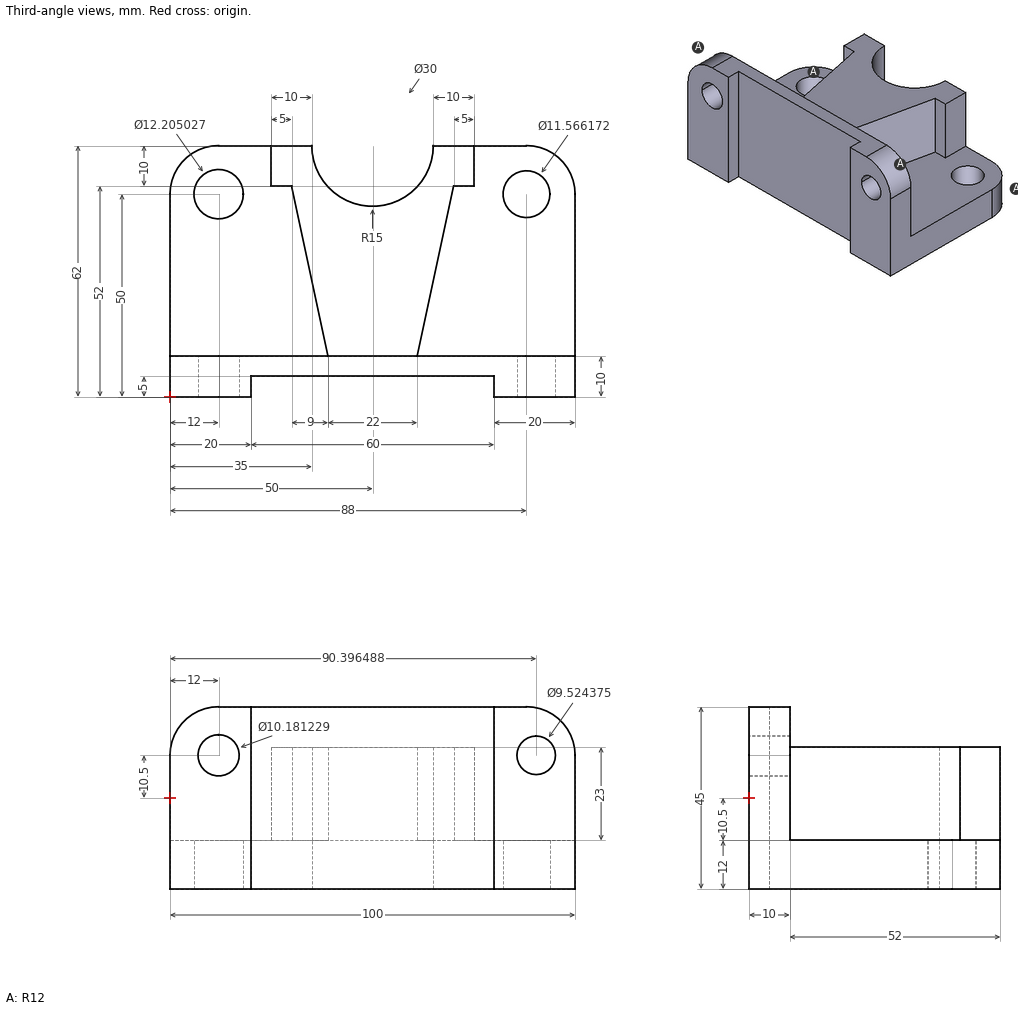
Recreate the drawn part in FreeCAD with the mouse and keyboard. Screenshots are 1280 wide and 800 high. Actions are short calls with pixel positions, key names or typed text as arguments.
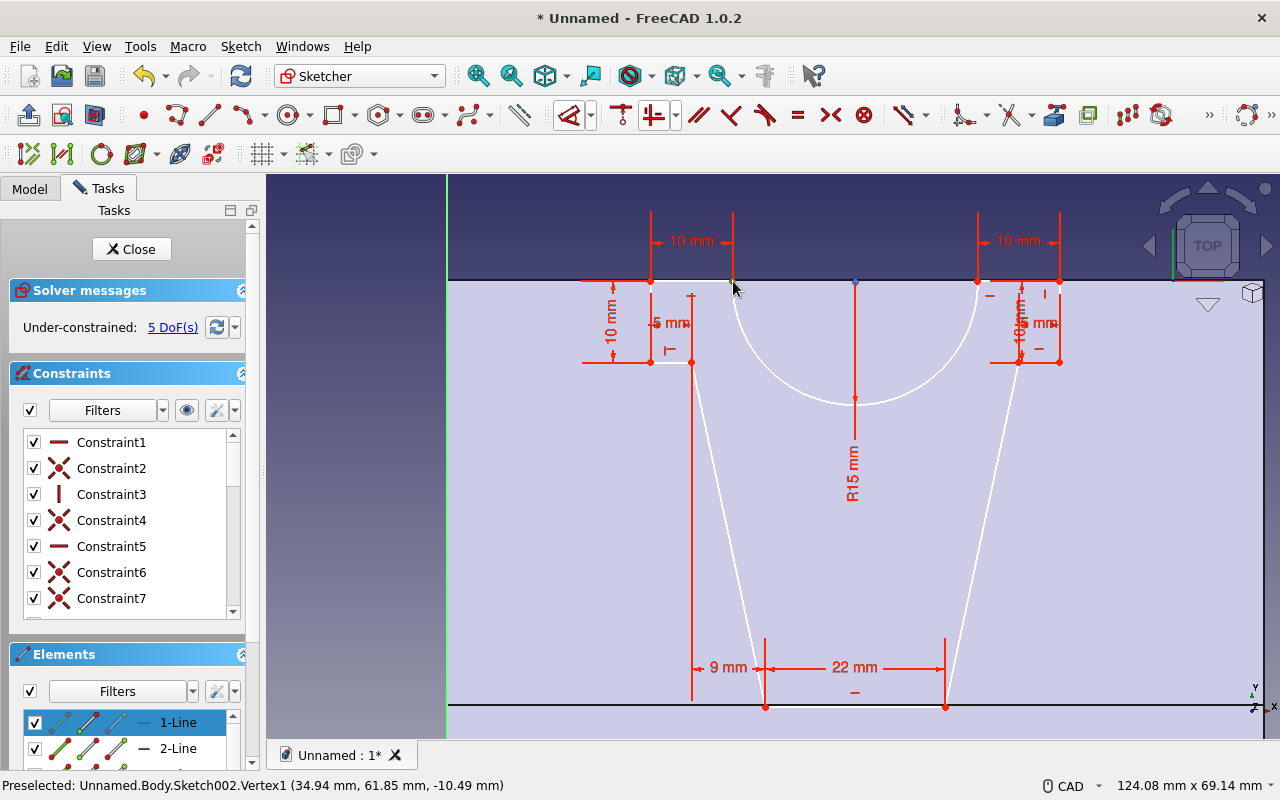
key(l)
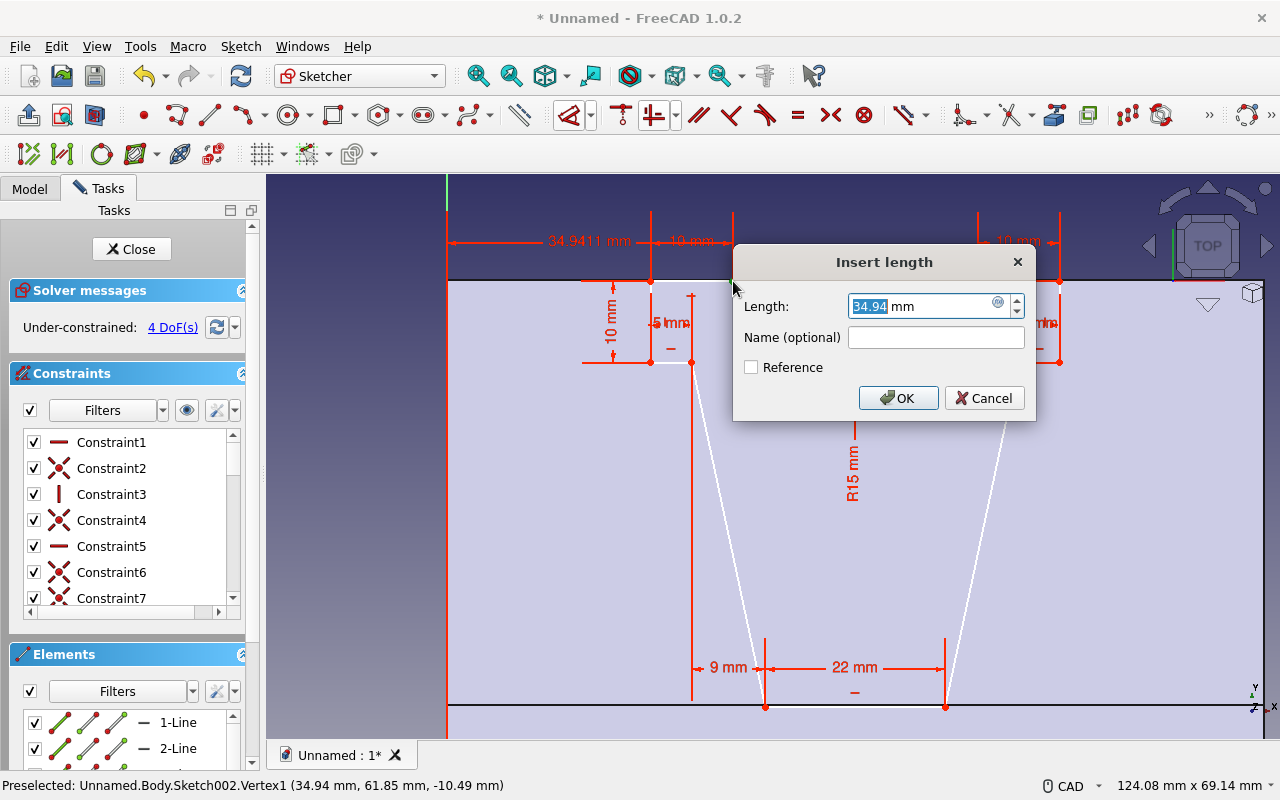
text(35)
key(Return)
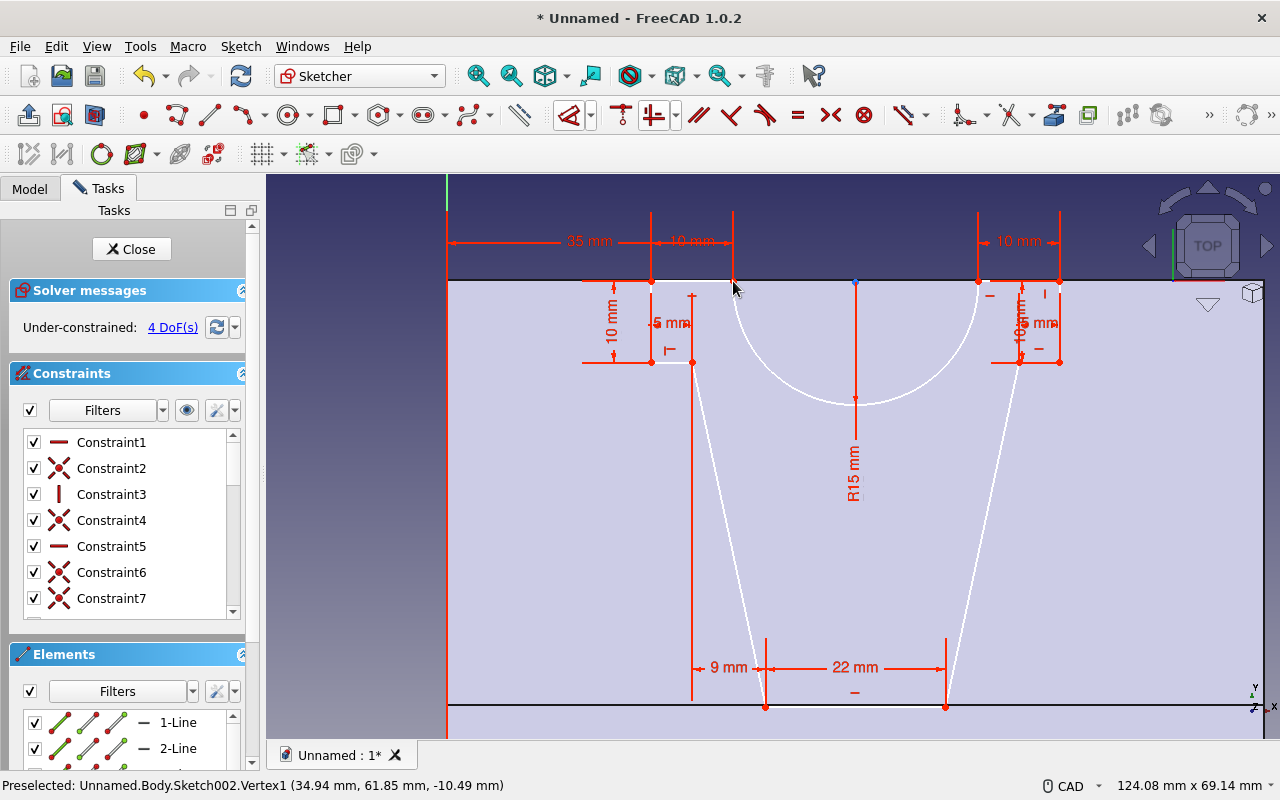
click(733, 281)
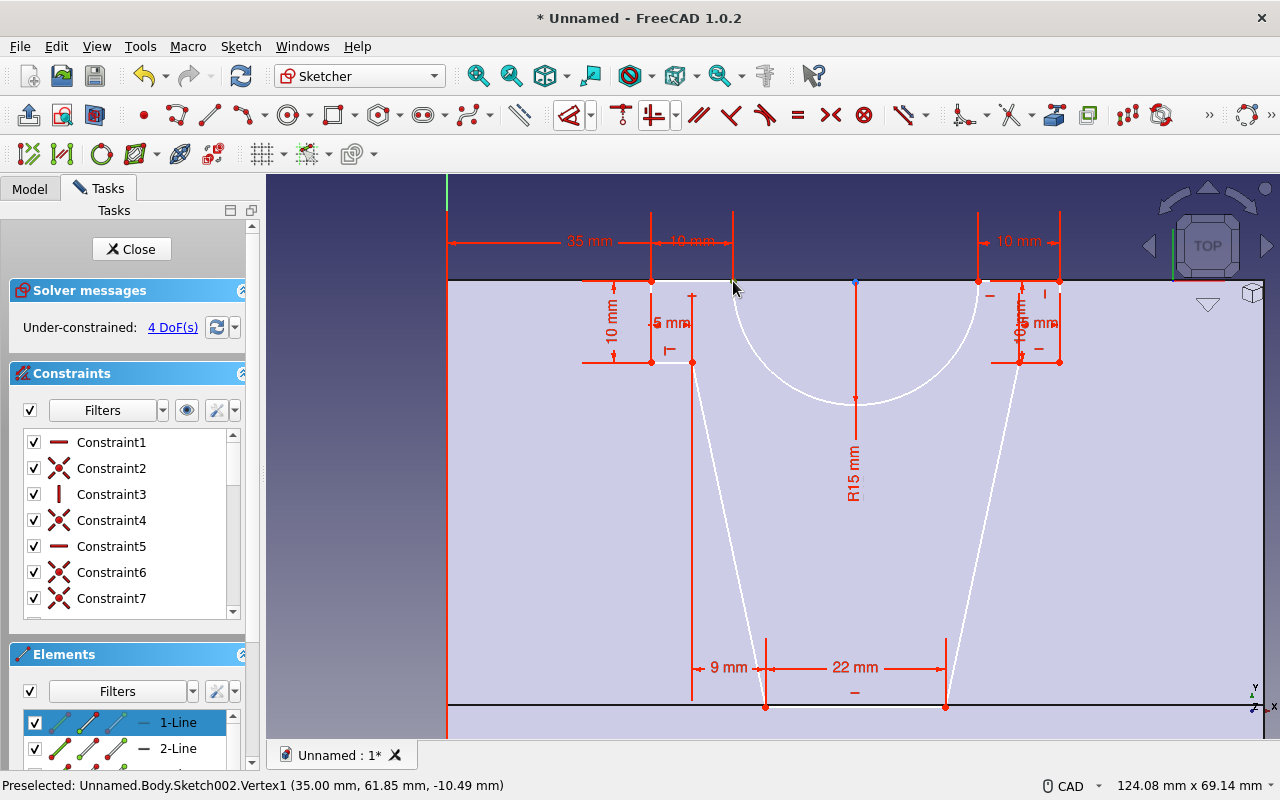
click(590, 116)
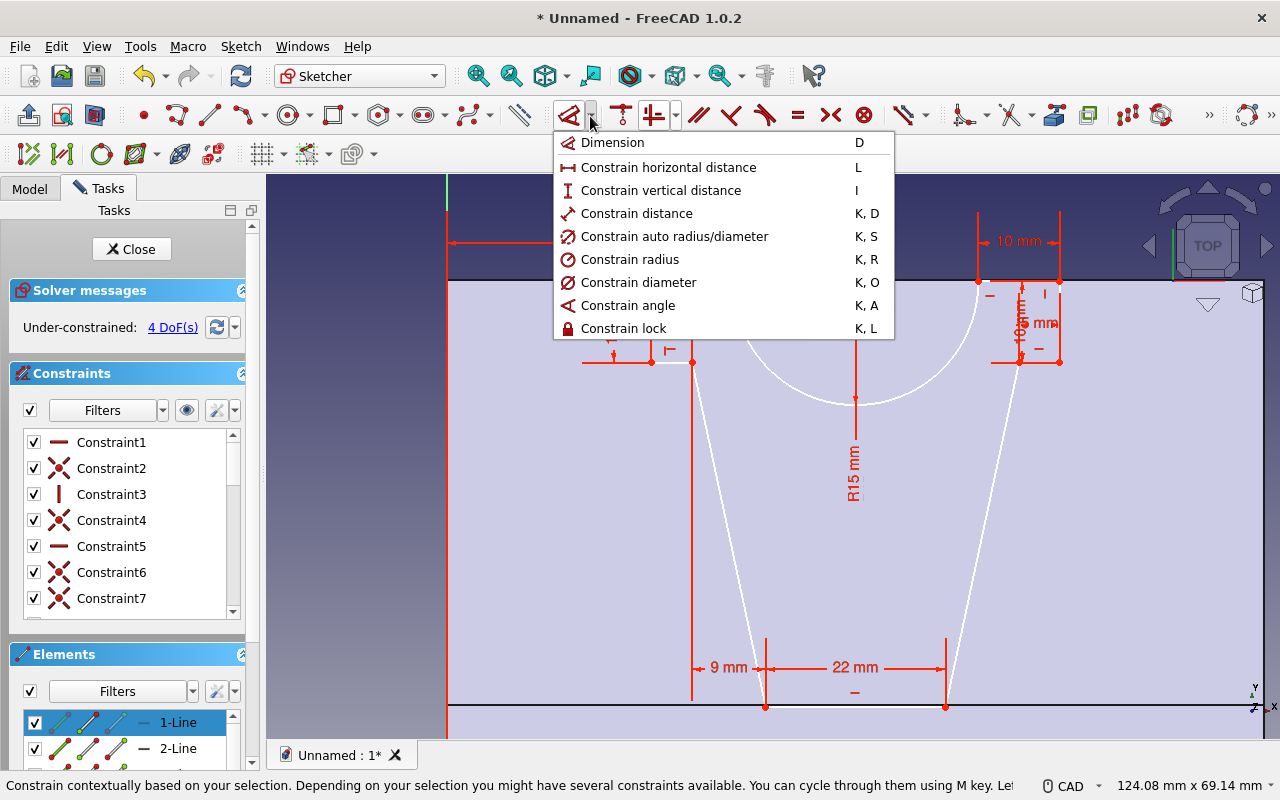
click(724, 190)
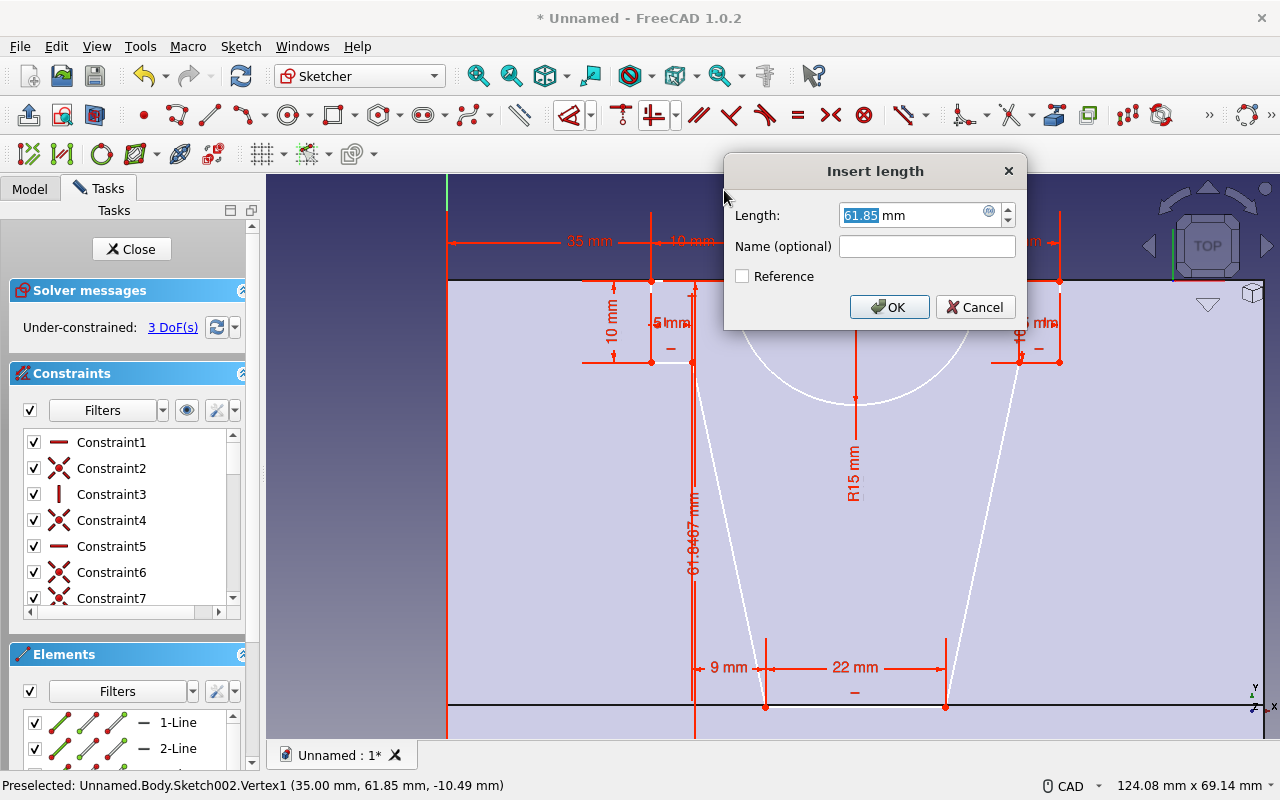
text(62)
key(Return)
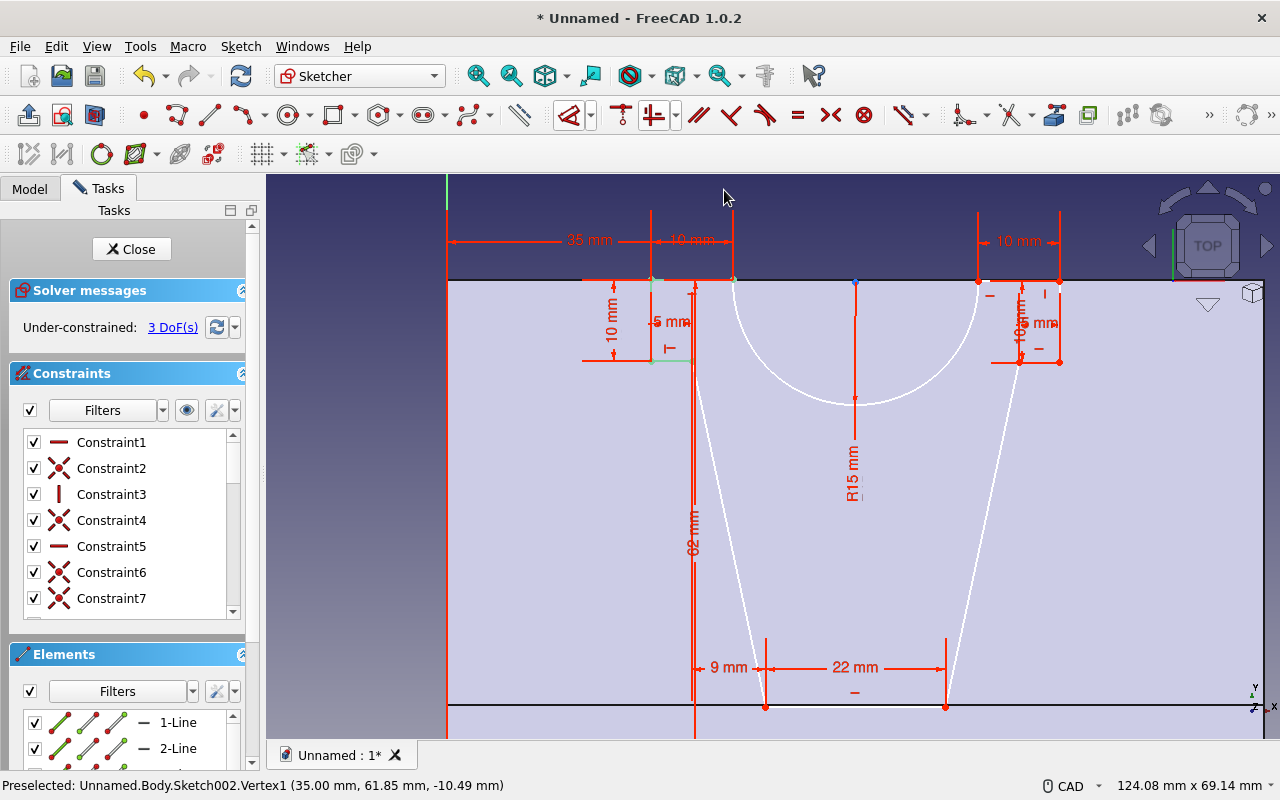
click(766, 707)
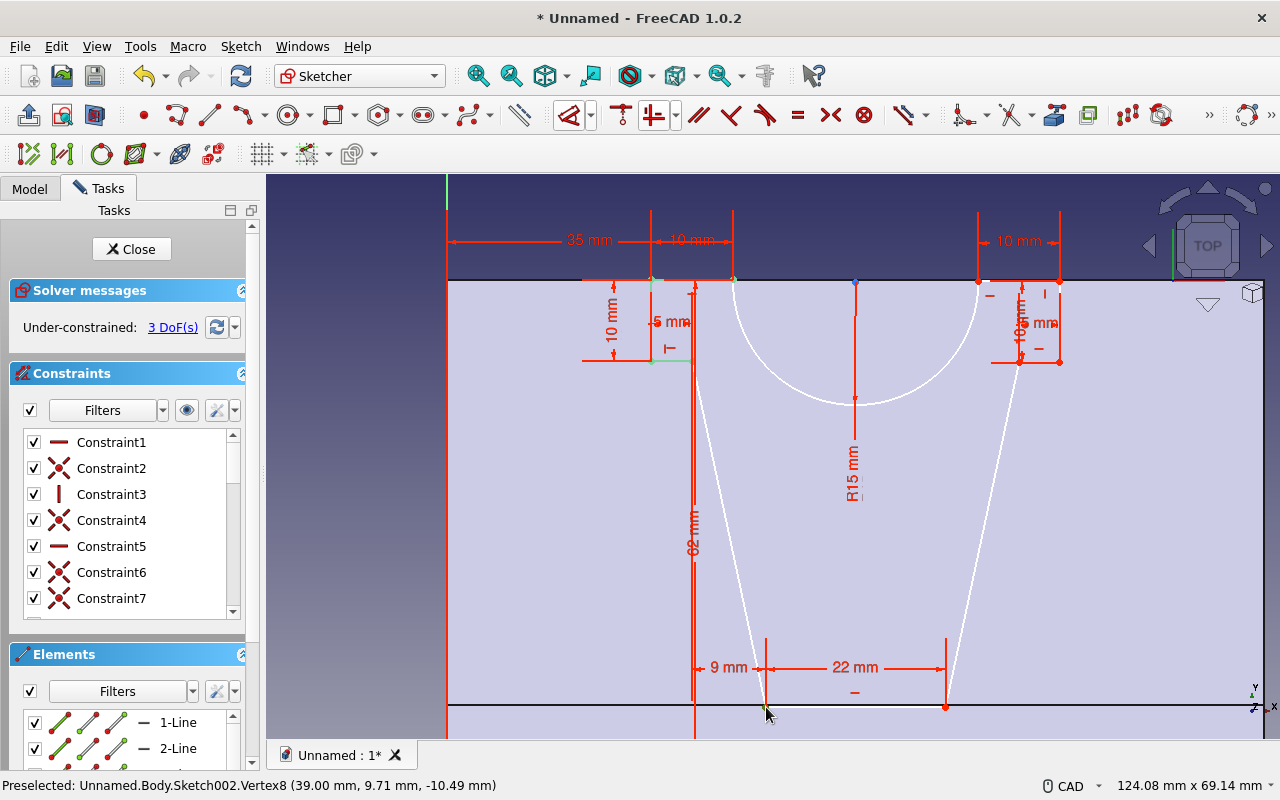
key(i)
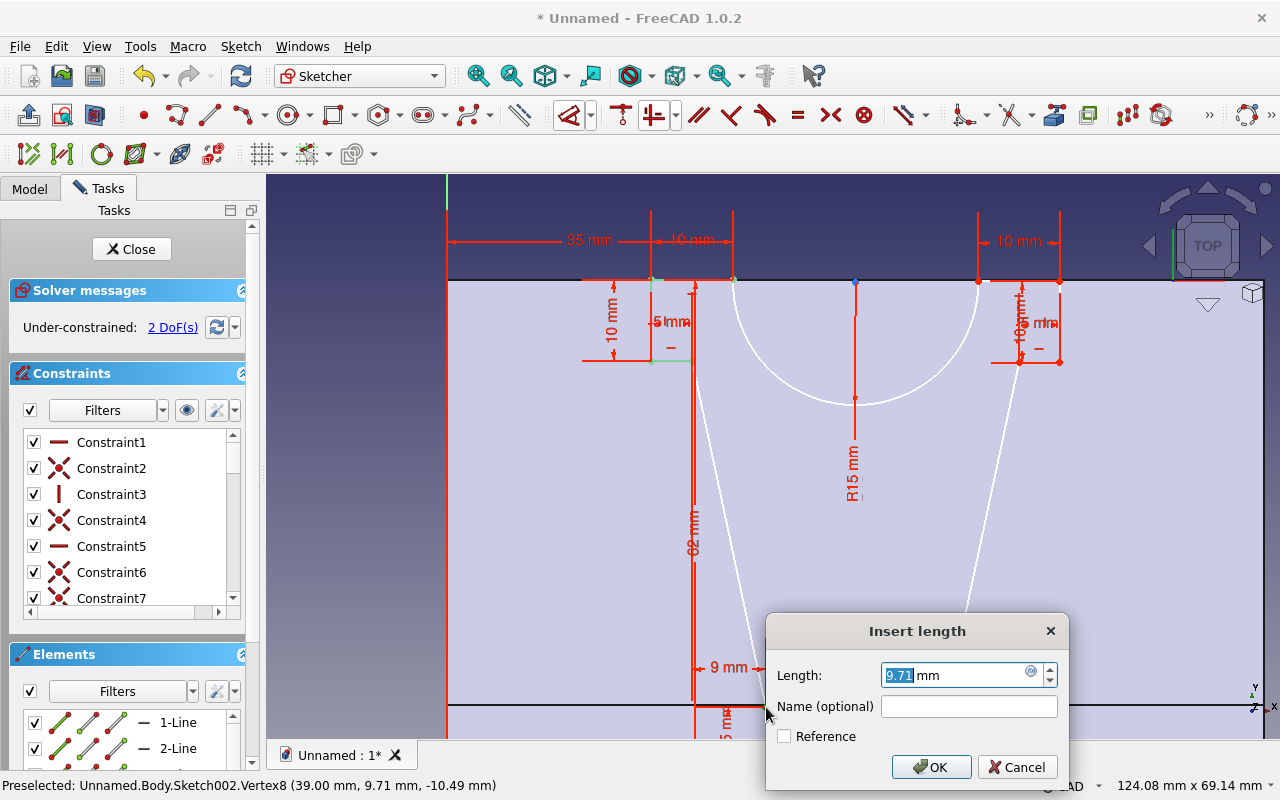
text(10)
key(Return)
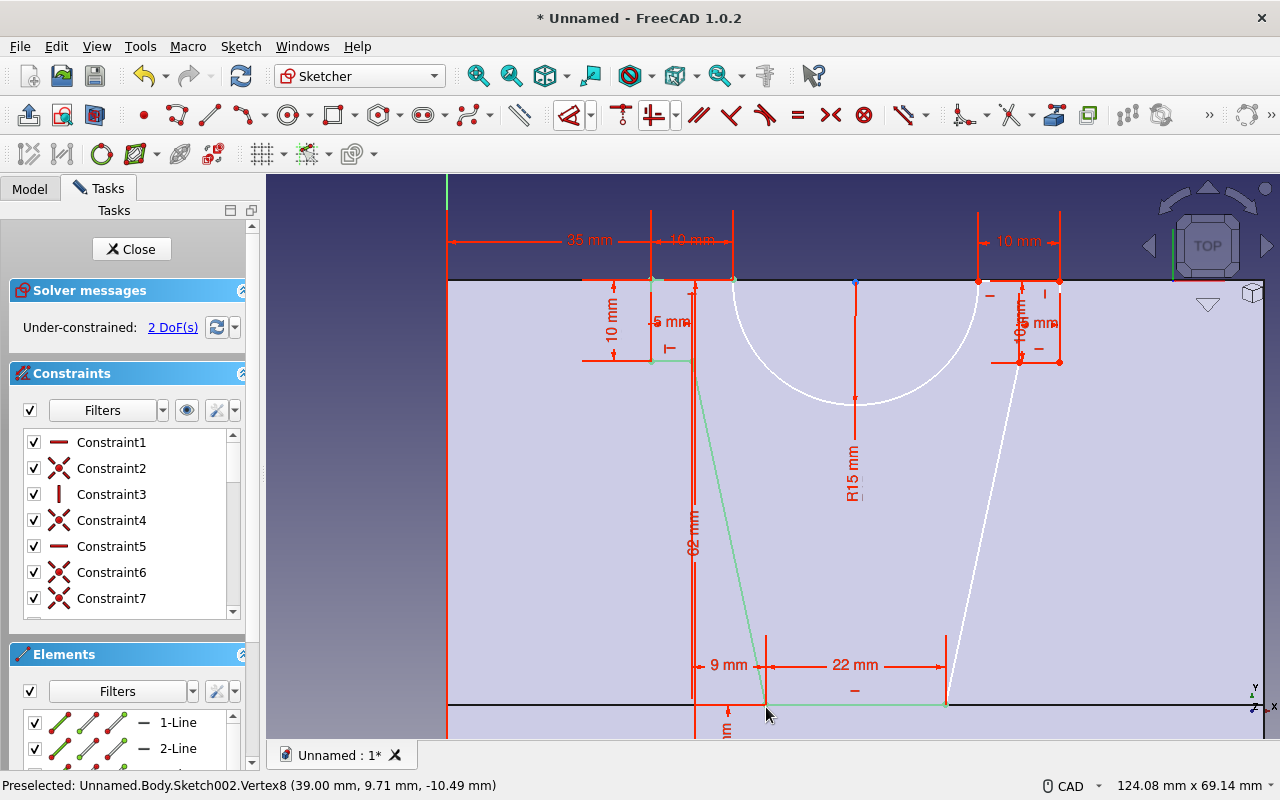
click(1019, 363)